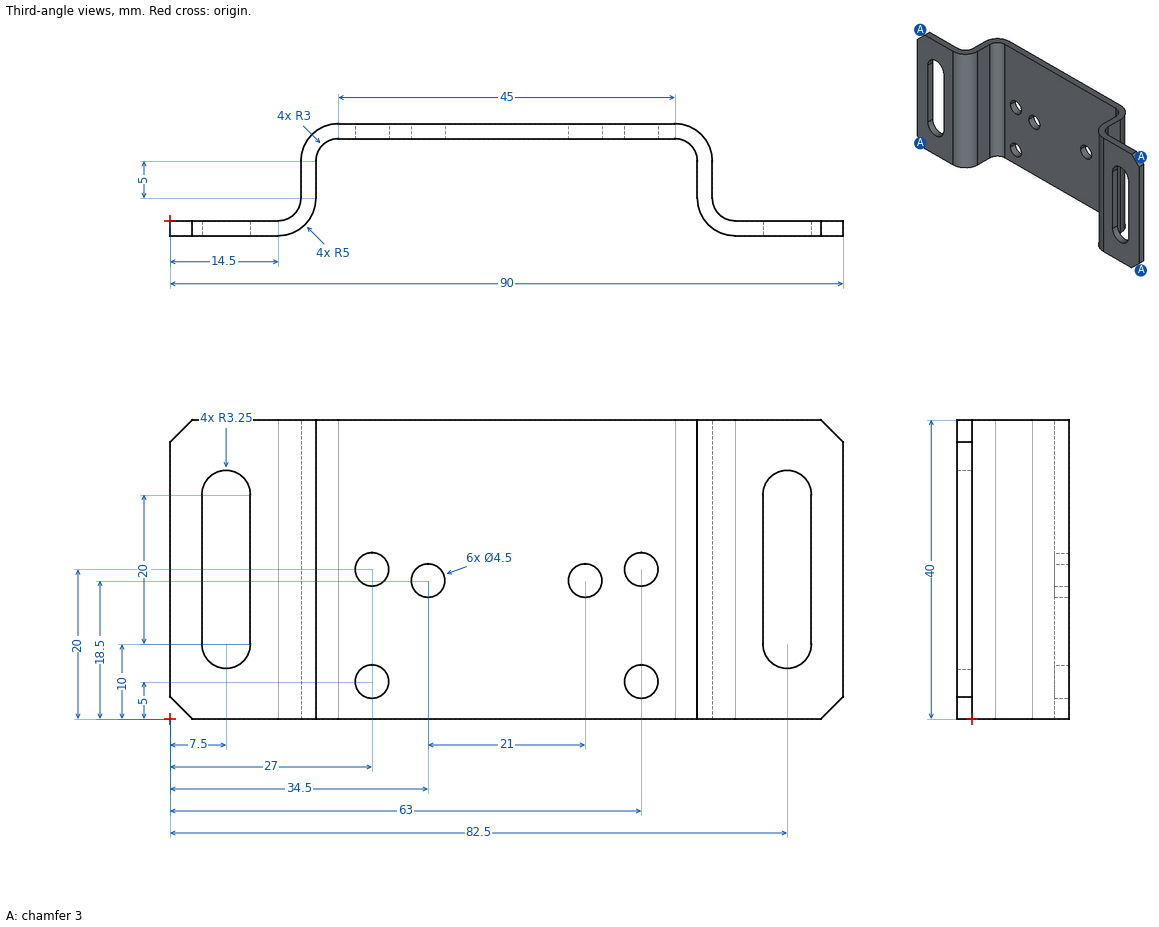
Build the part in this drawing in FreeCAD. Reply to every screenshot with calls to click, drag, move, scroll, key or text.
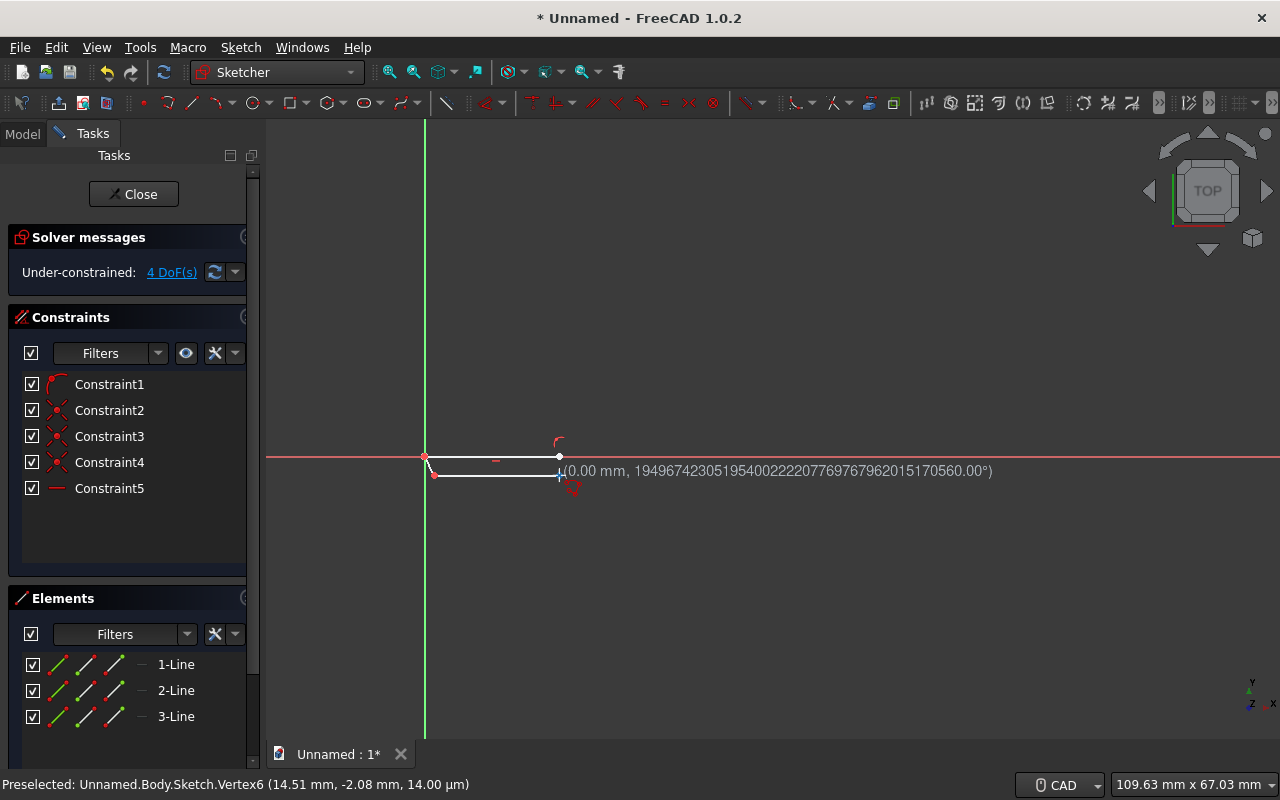
key(g)
key(l)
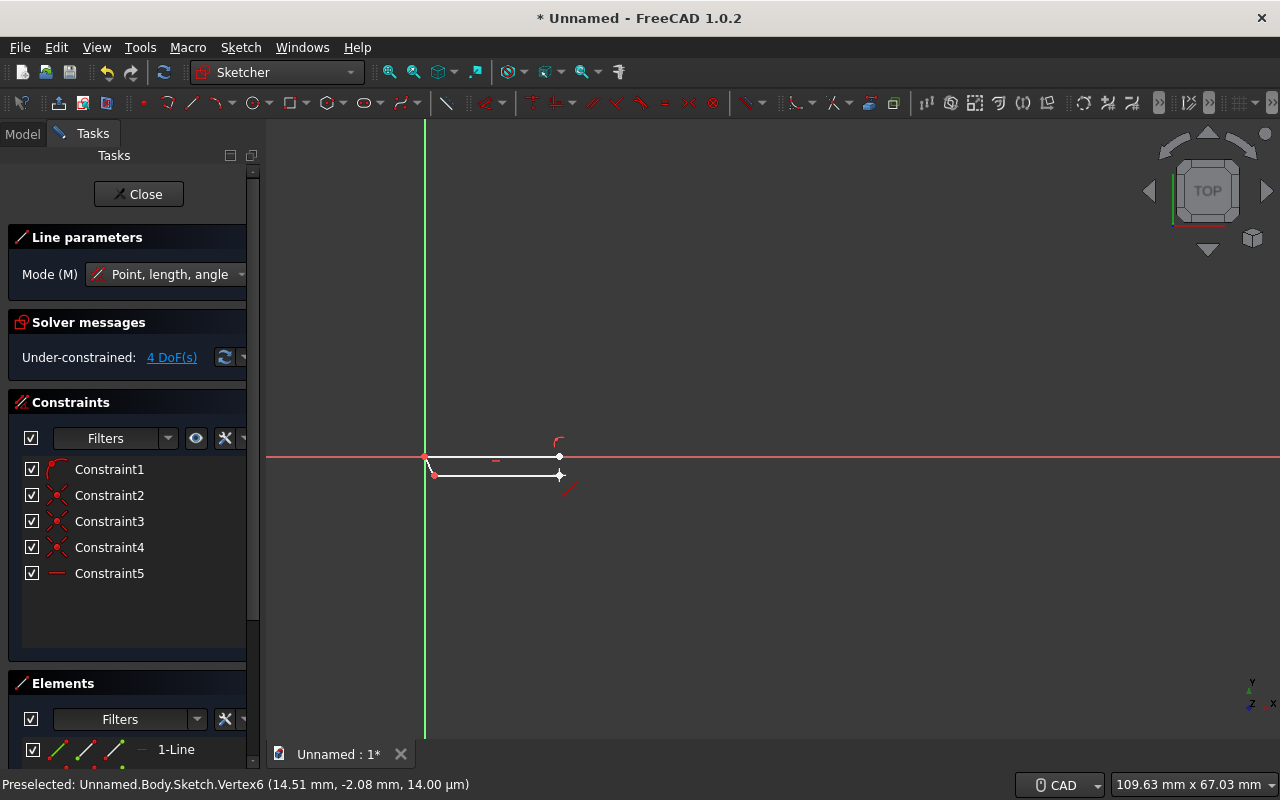
click(605, 429)
click(605, 383)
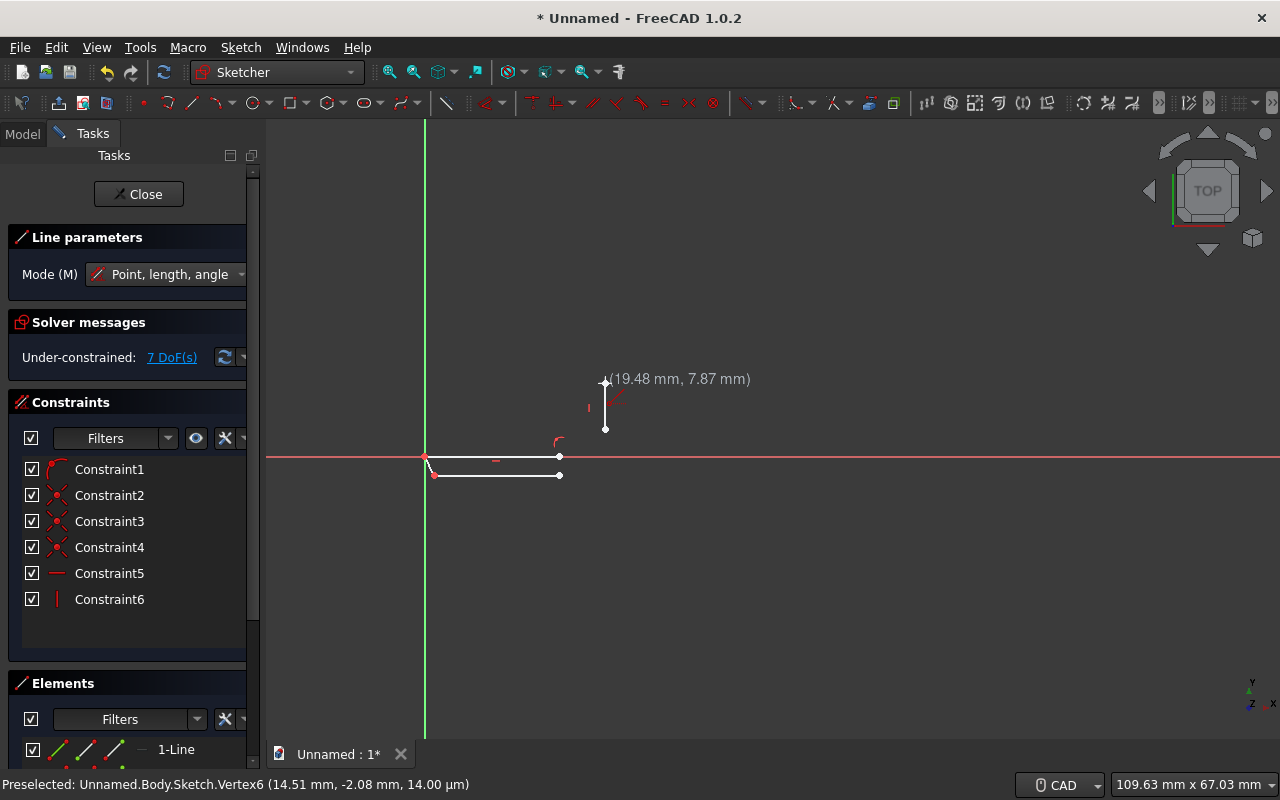
click(633, 355)
click(1049, 355)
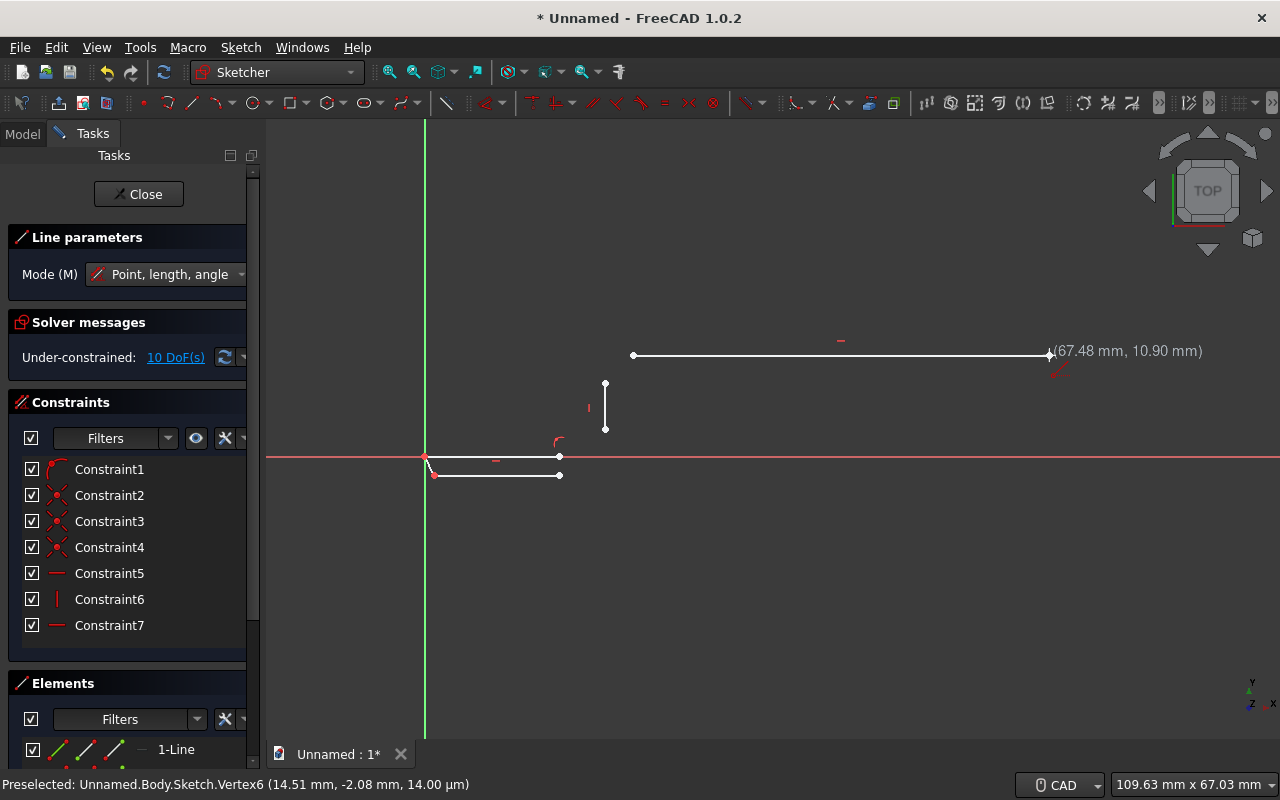
click(1077, 383)
click(1077, 429)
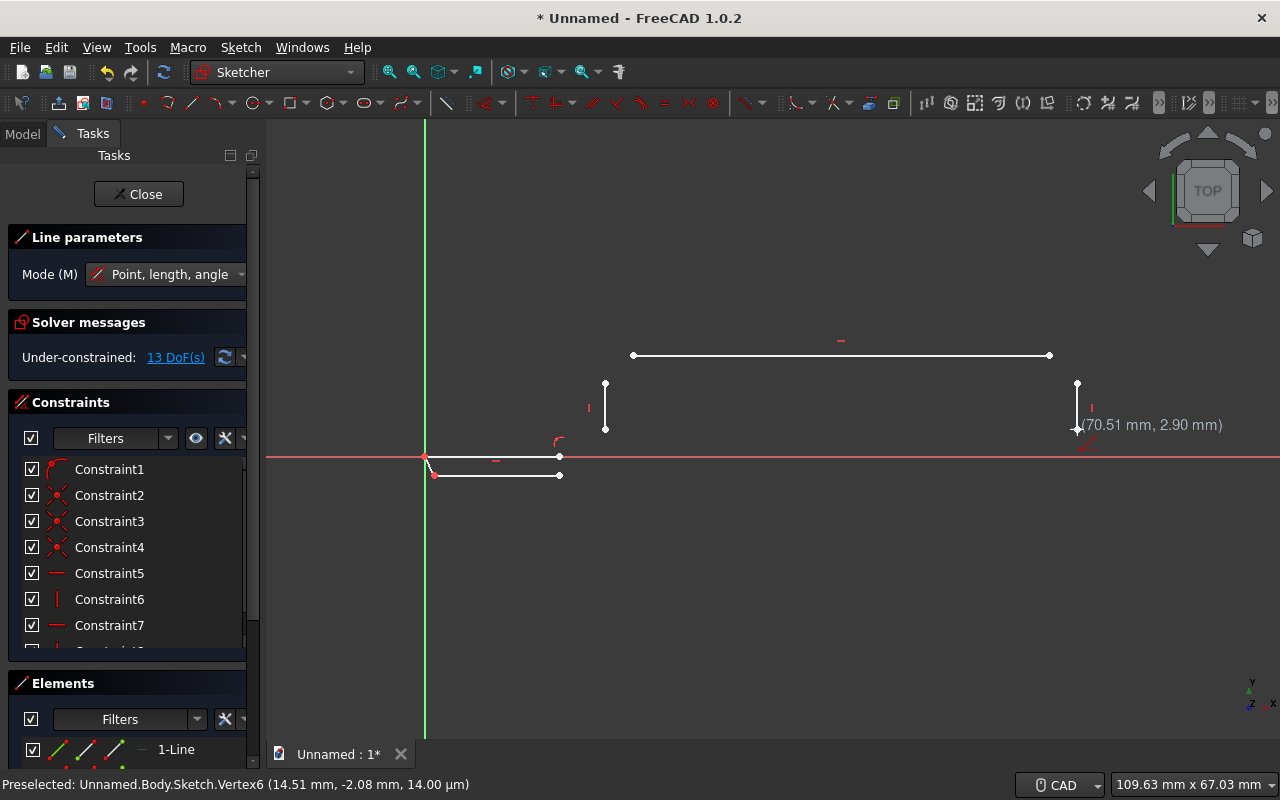
key(g)
key(m)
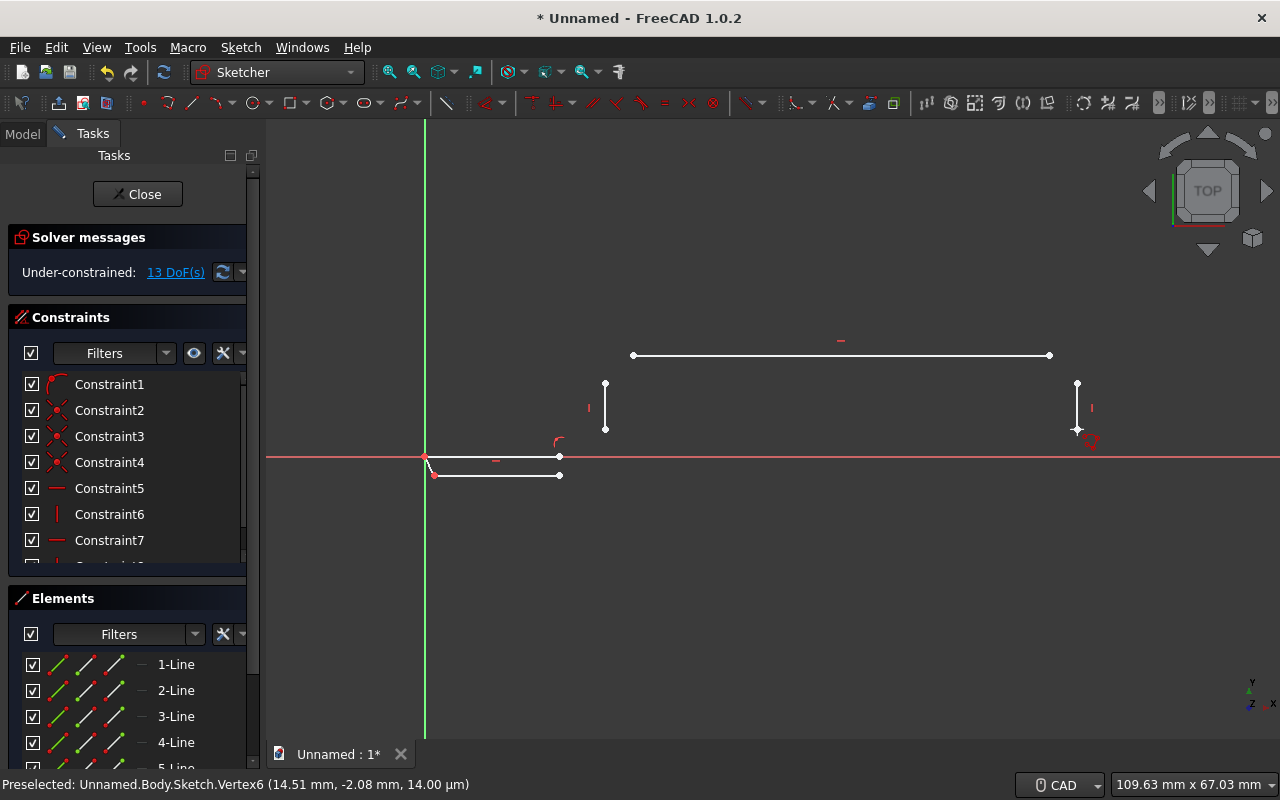
scroll(427, 476, down, 2)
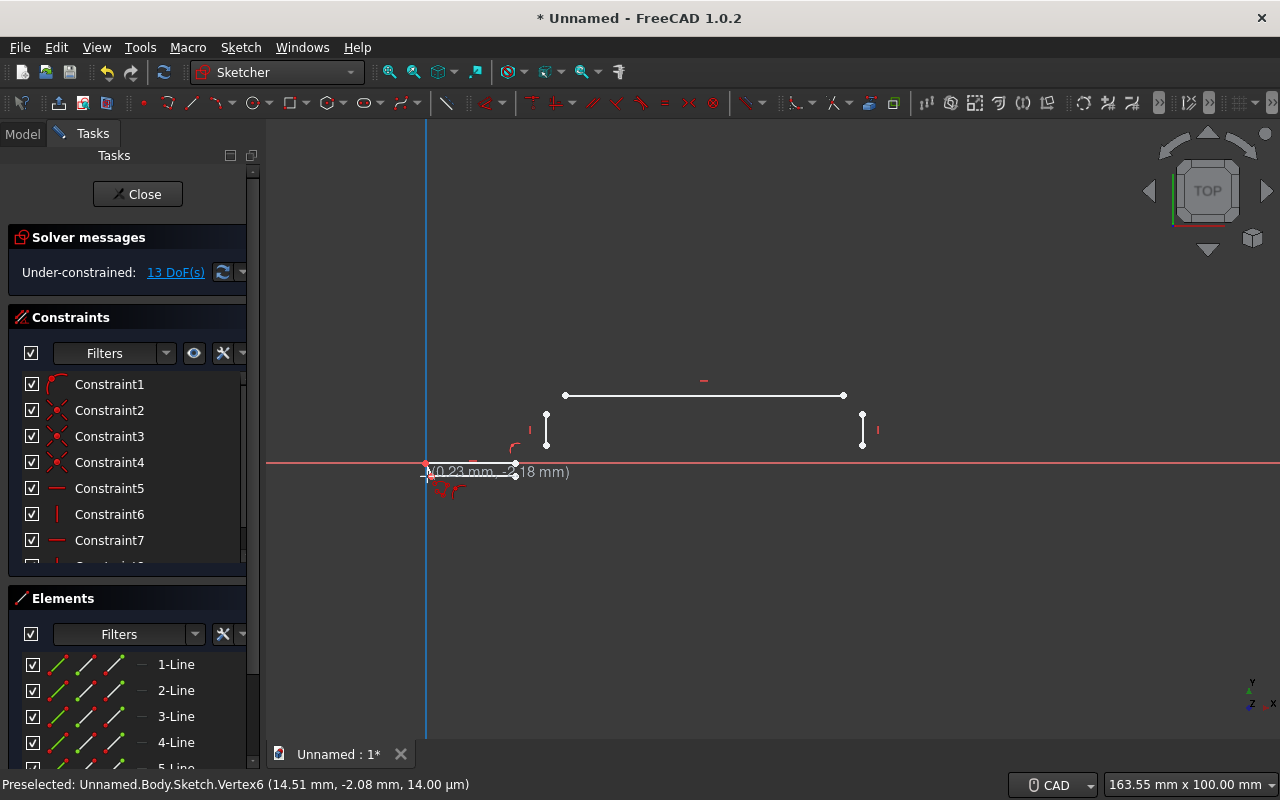
scroll(894, 476, up, 2)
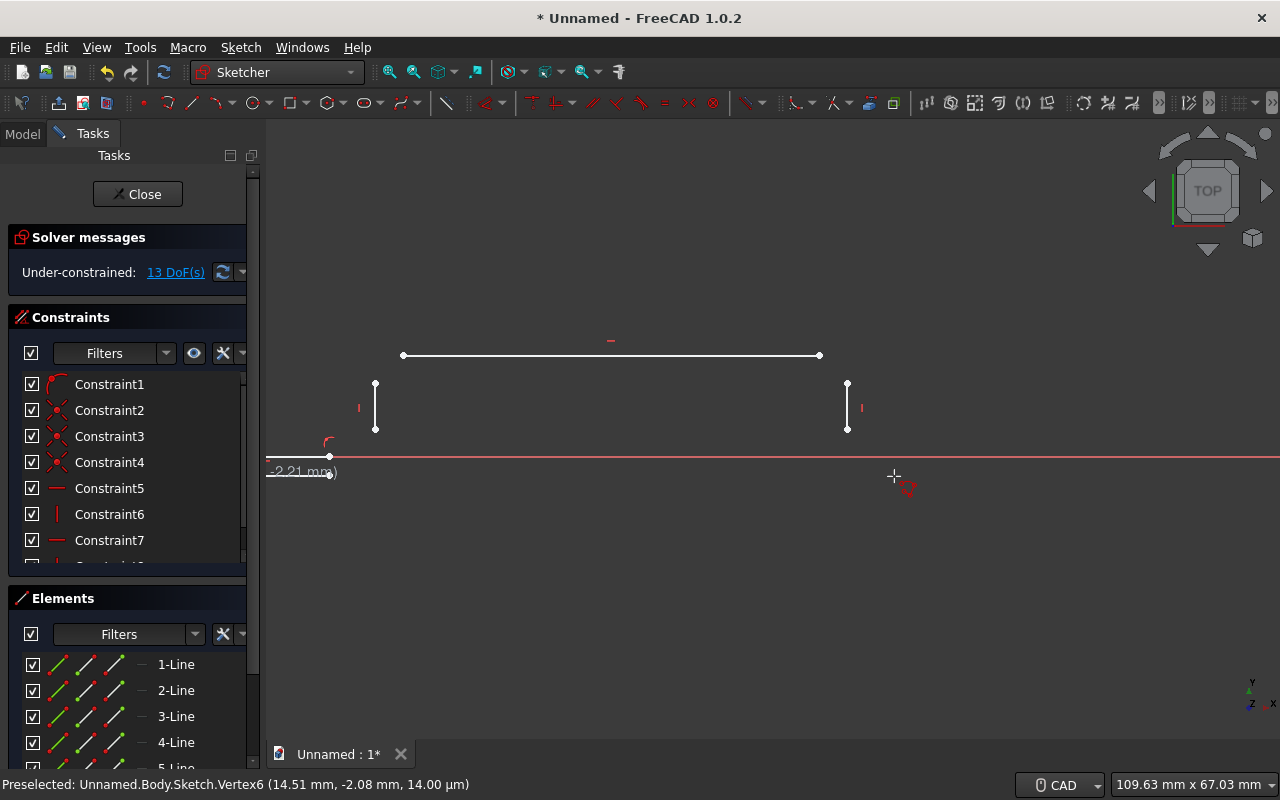
click(893, 475)
click(1027, 475)
click(1027, 457)
click(893, 448)
right_click(893, 448)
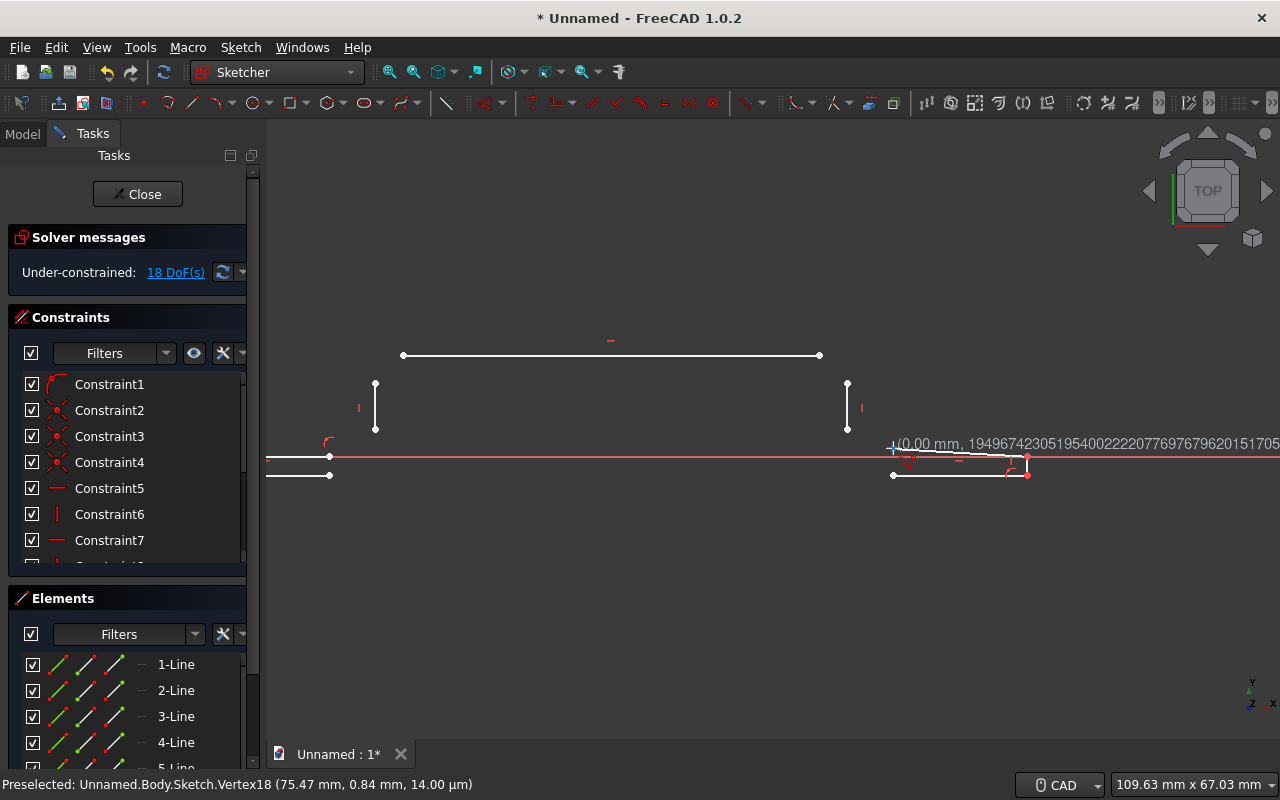
click(192, 104)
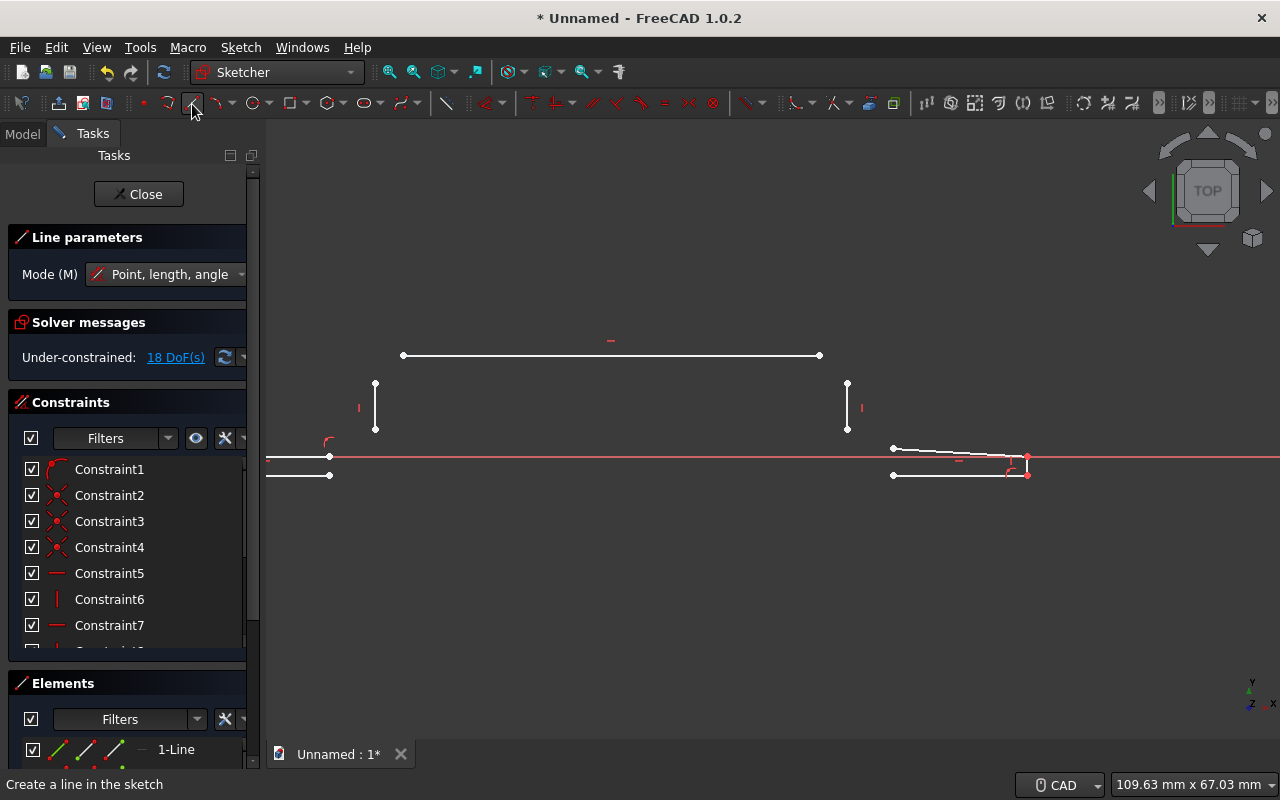
click(865, 429)
click(865, 383)